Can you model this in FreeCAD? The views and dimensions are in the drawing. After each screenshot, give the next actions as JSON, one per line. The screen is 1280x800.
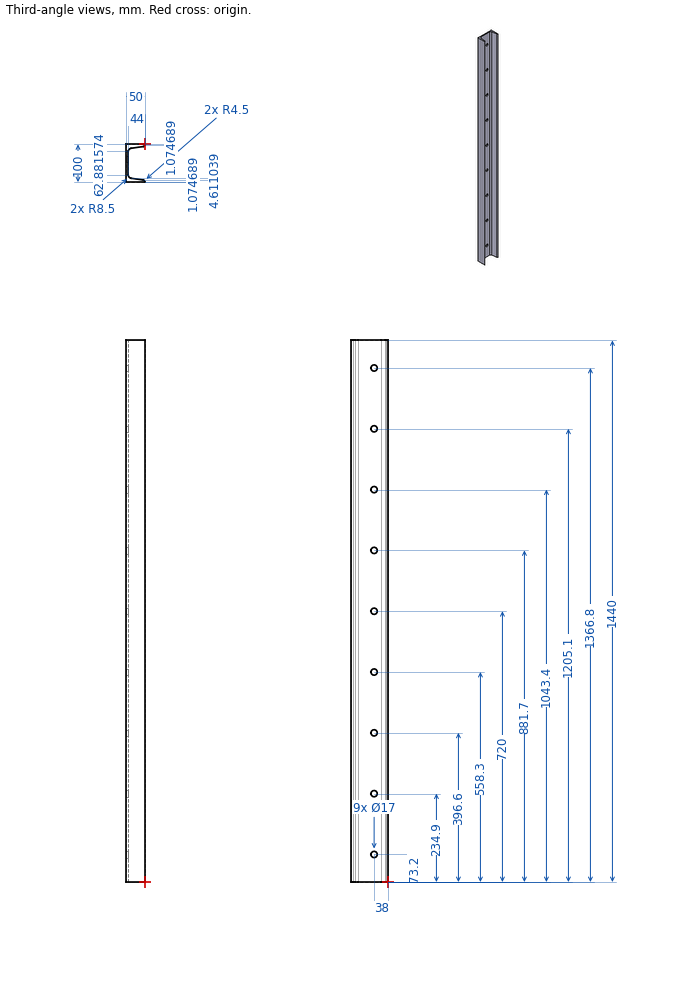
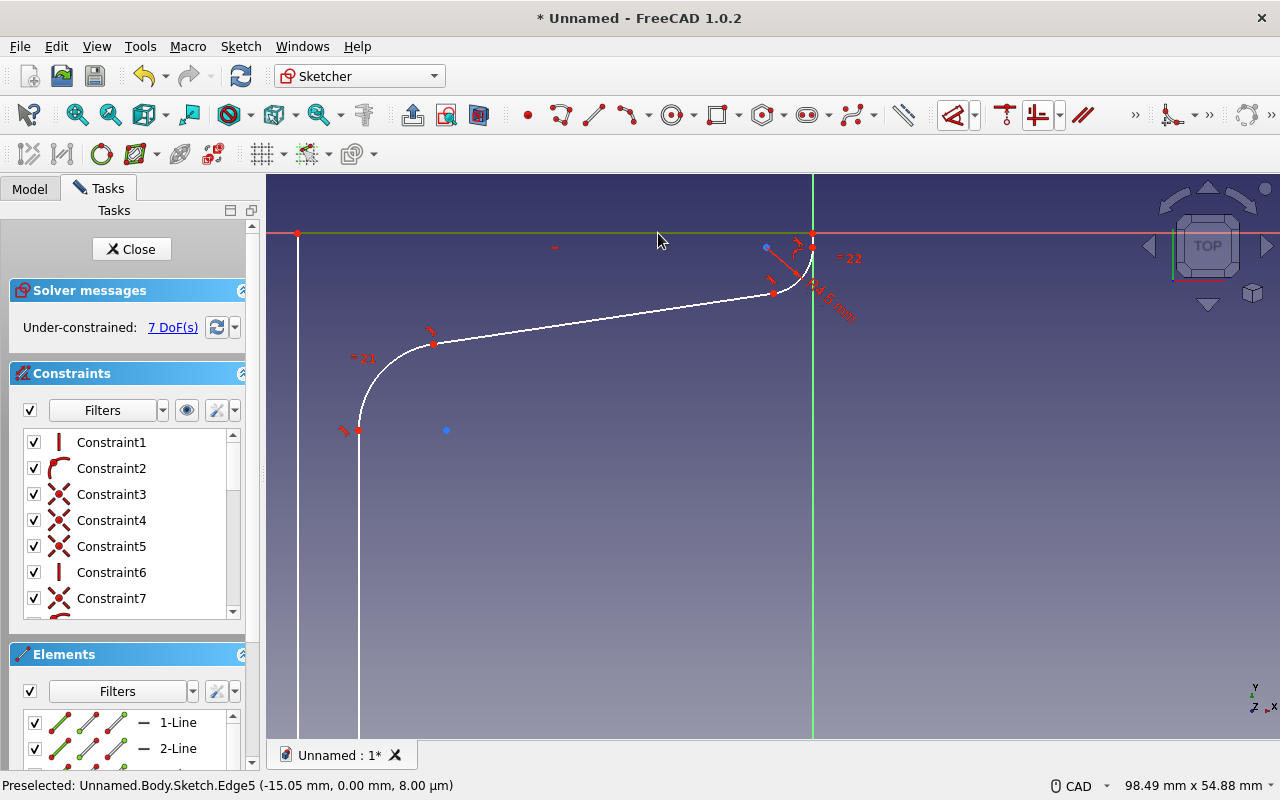
{"action": "left_click", "coordinate": [974, 116]}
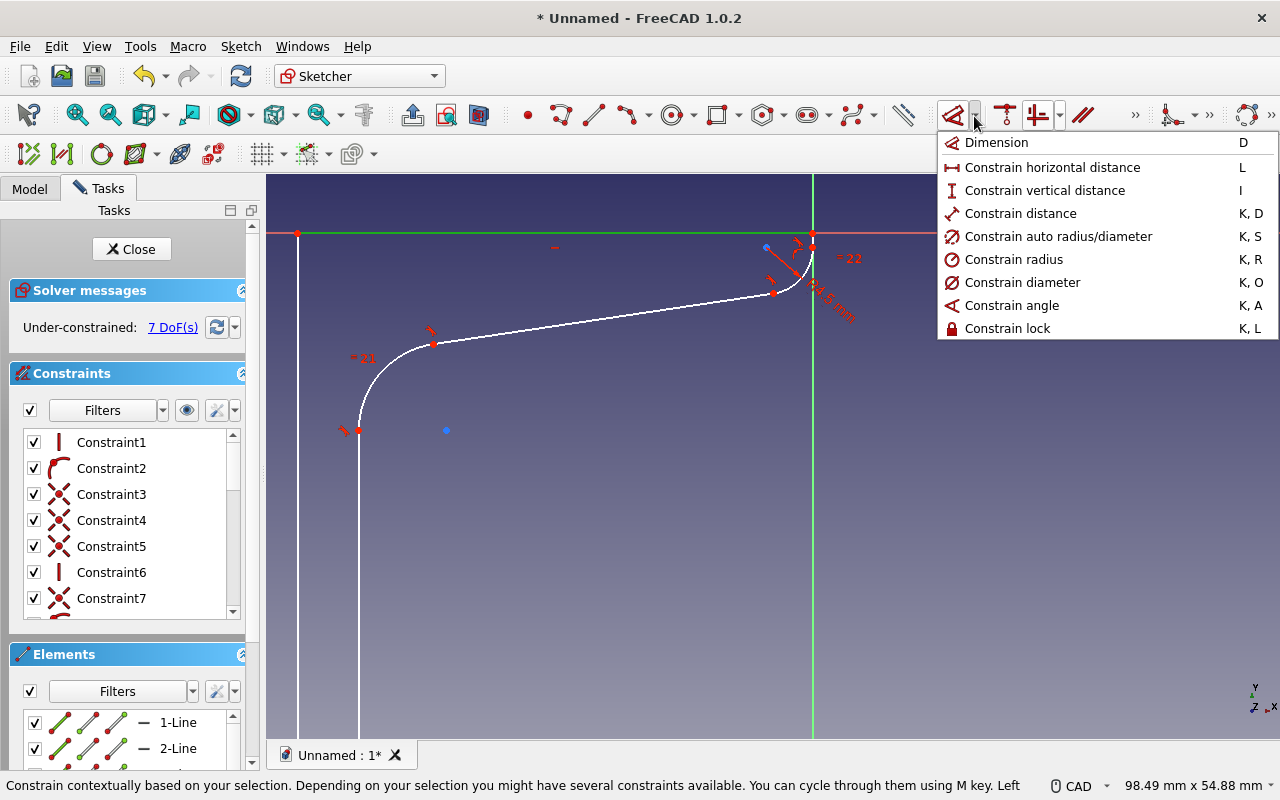
{"action": "left_click", "coordinate": [1108, 168]}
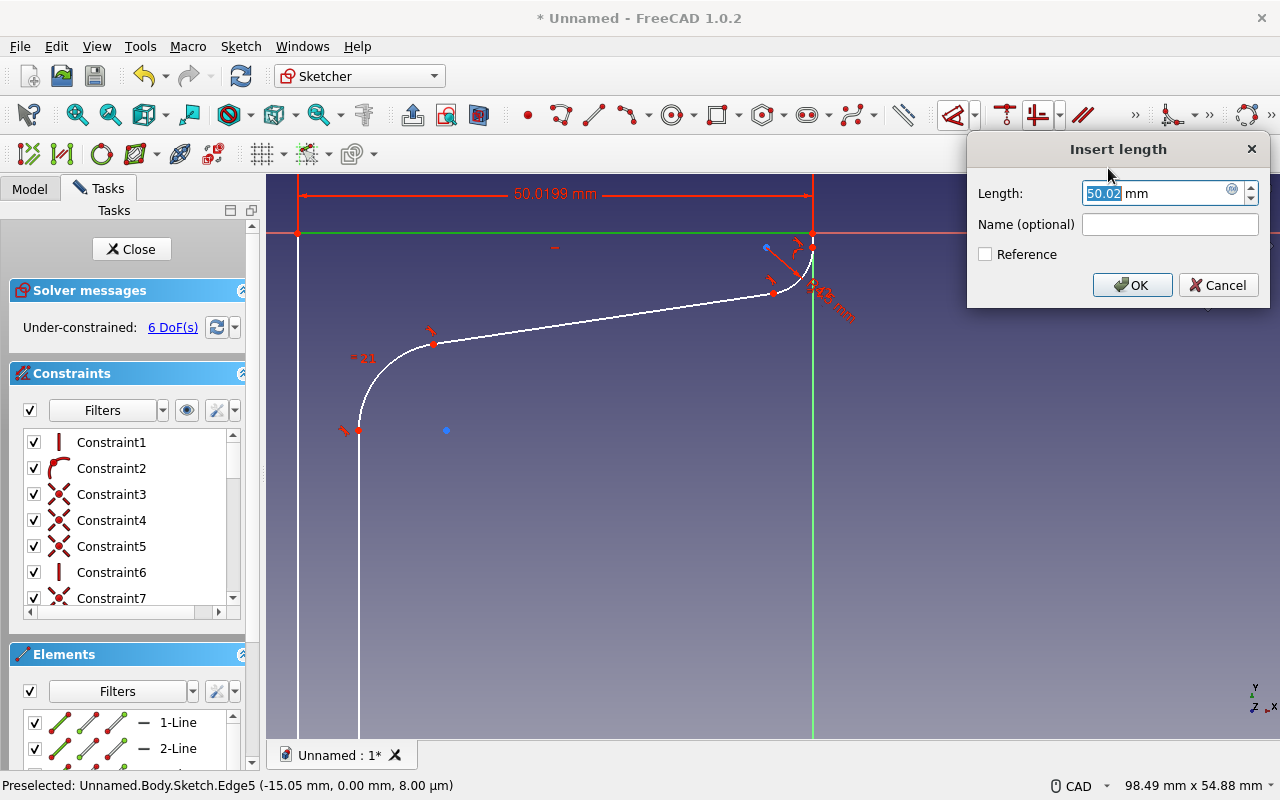
{"action": "type", "text": "50"}
{"action": "key", "text": "Return"}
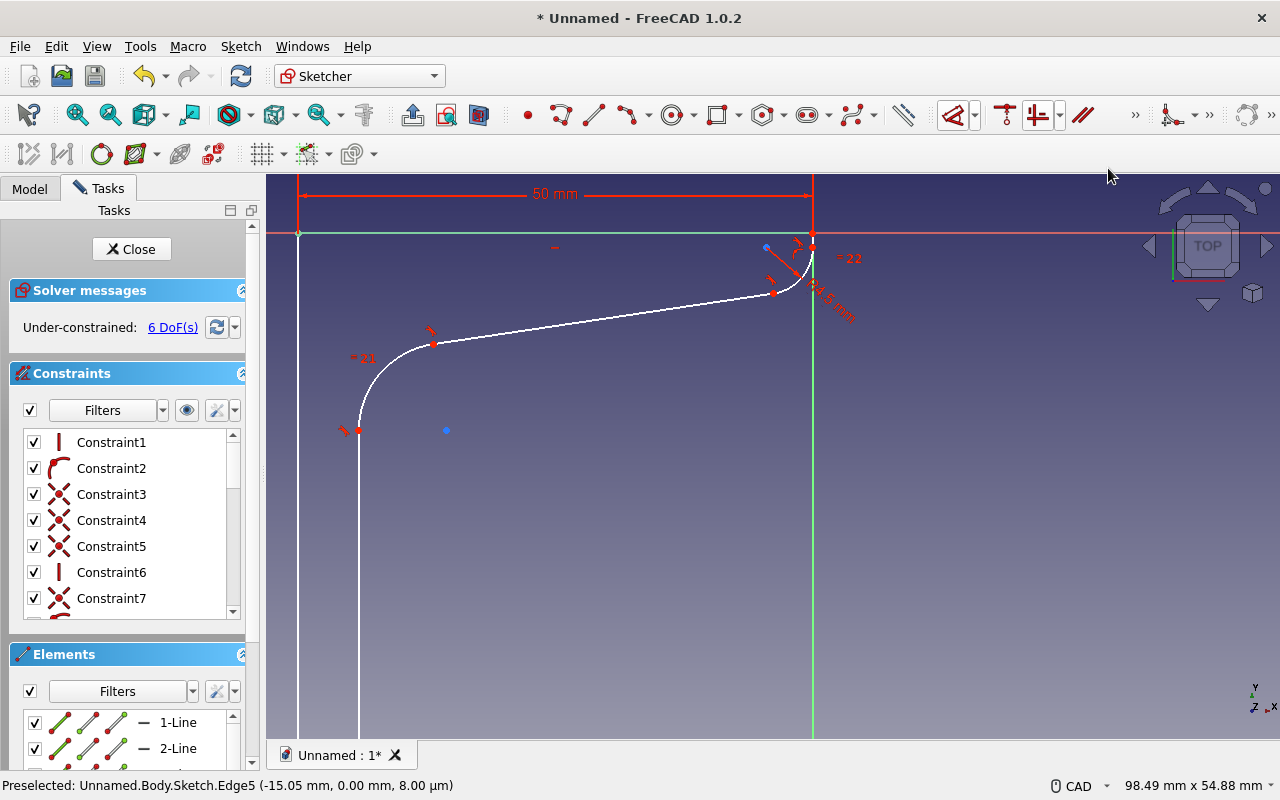
{"action": "left_click", "coordinate": [298, 543]}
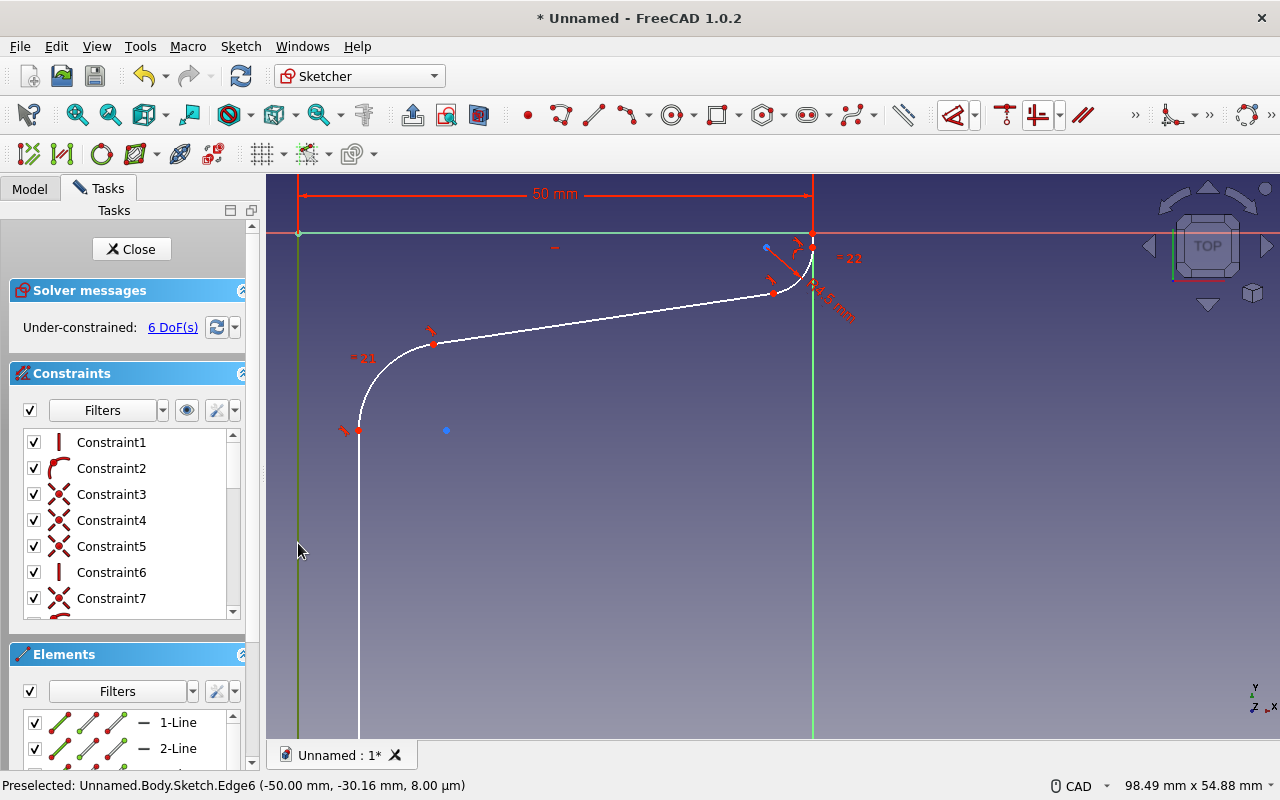
{"action": "left_click", "coordinate": [974, 116]}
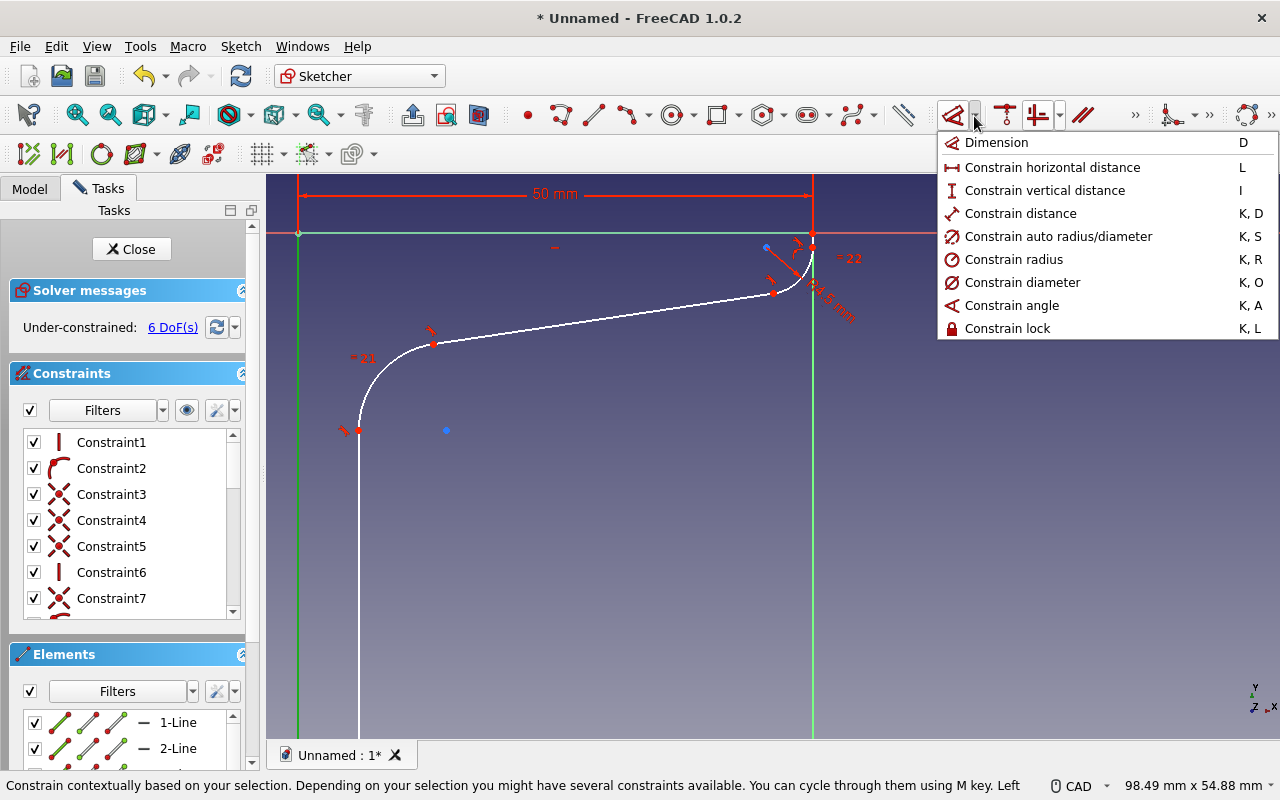
{"action": "left_click", "coordinate": [1108, 190]}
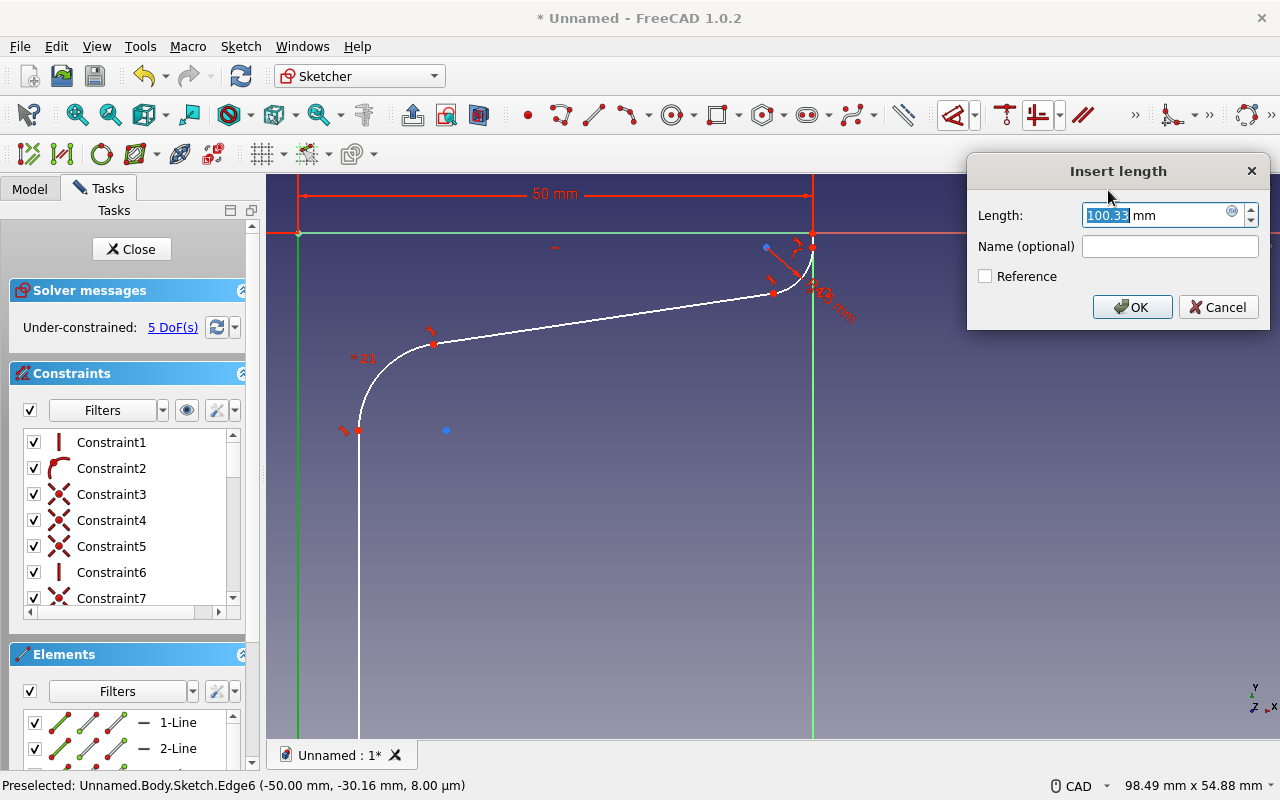
{"action": "type", "text": "100"}
{"action": "key", "text": "Return"}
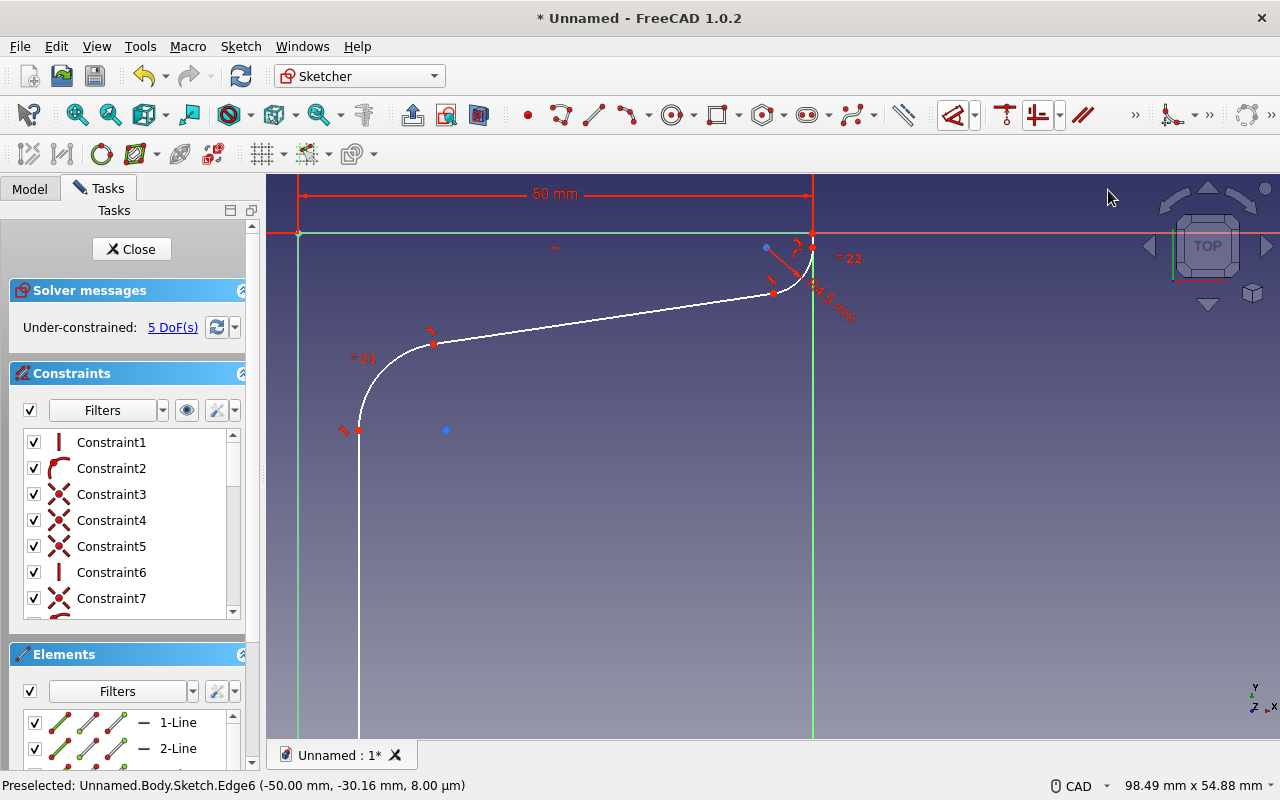
{"action": "scroll", "coordinate": [791, 287], "scroll_direction": "down", "scroll_amount": 5}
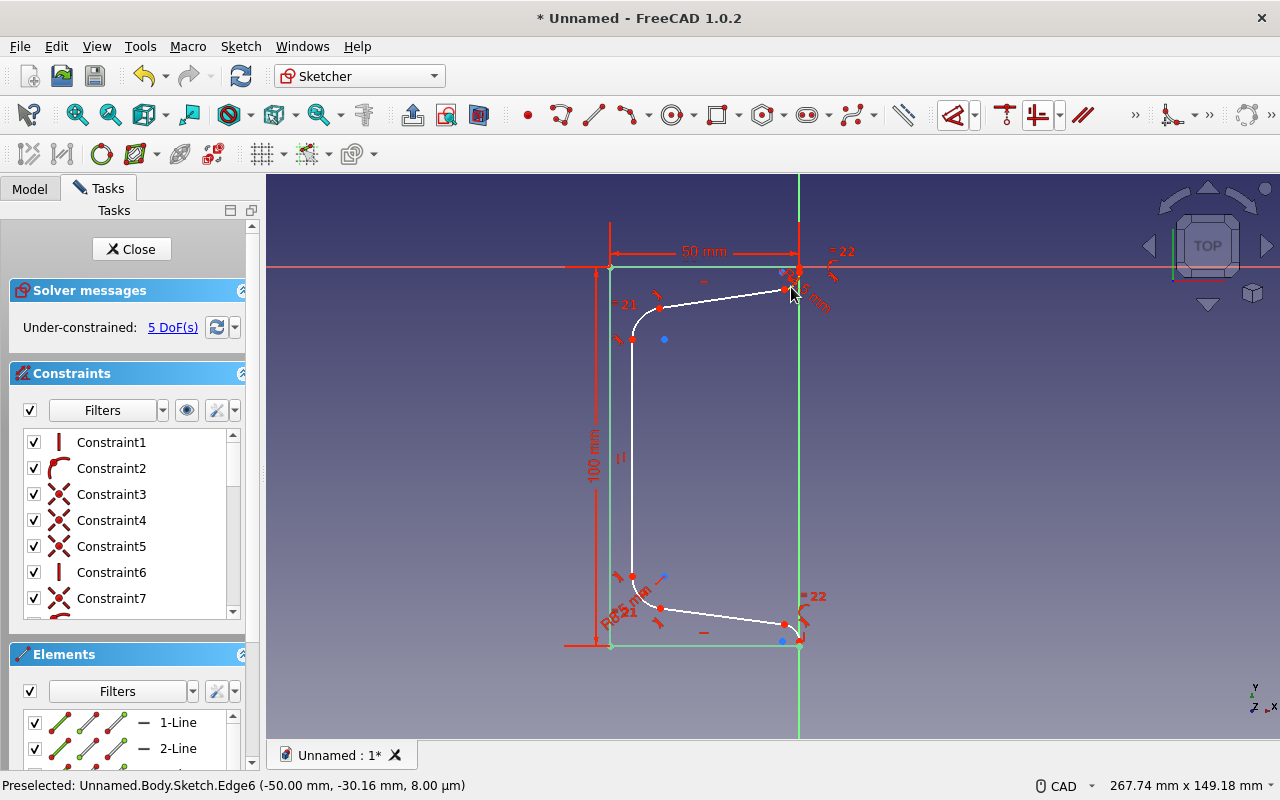
{"action": "left_click", "coordinate": [632, 577]}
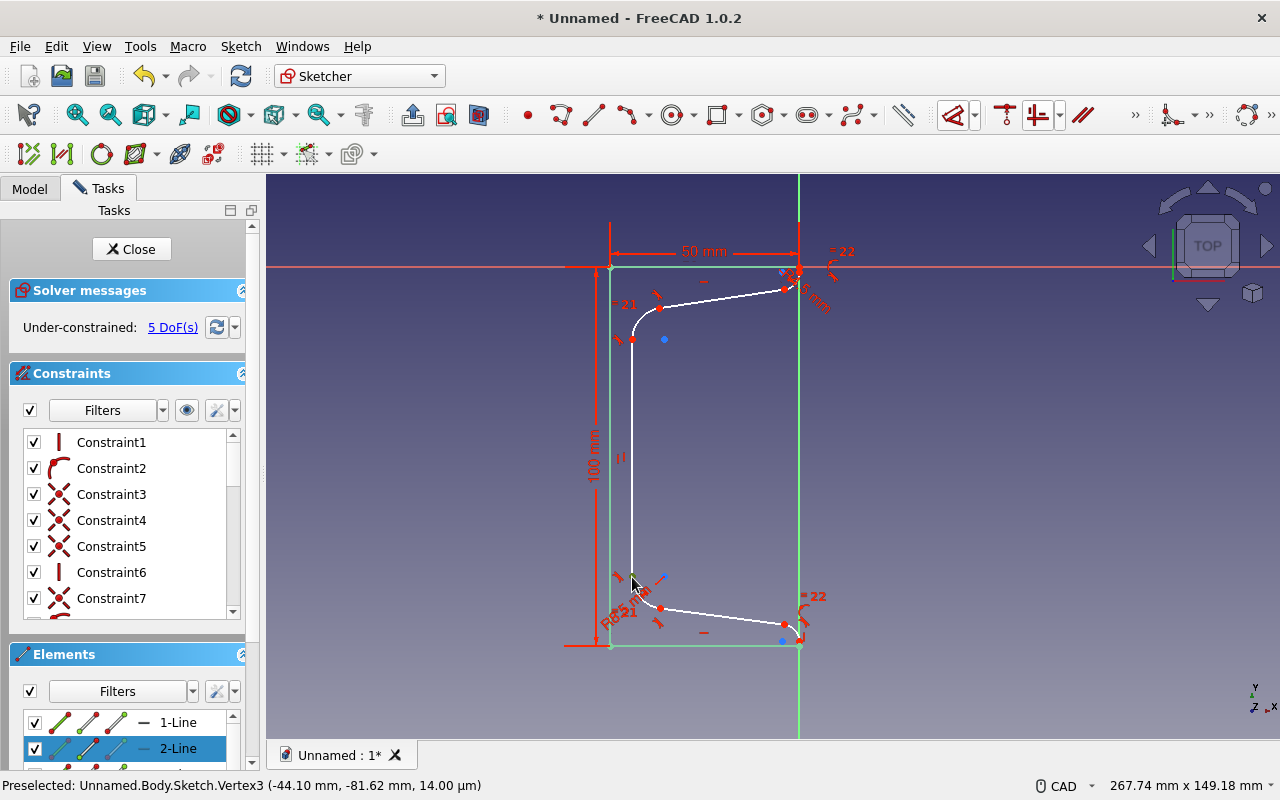
{"action": "left_click", "coordinate": [974, 116]}